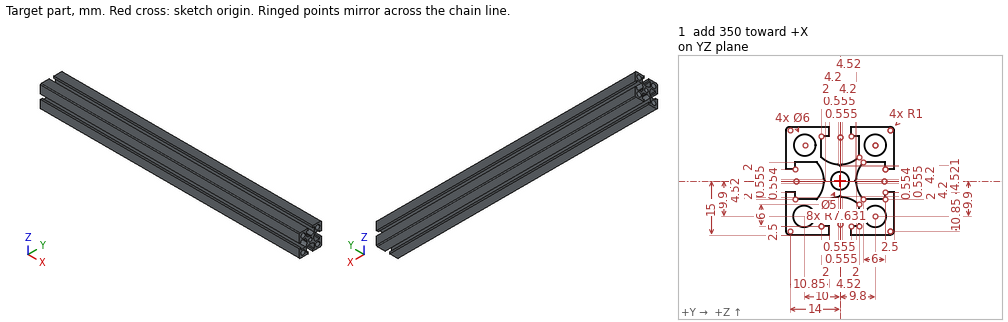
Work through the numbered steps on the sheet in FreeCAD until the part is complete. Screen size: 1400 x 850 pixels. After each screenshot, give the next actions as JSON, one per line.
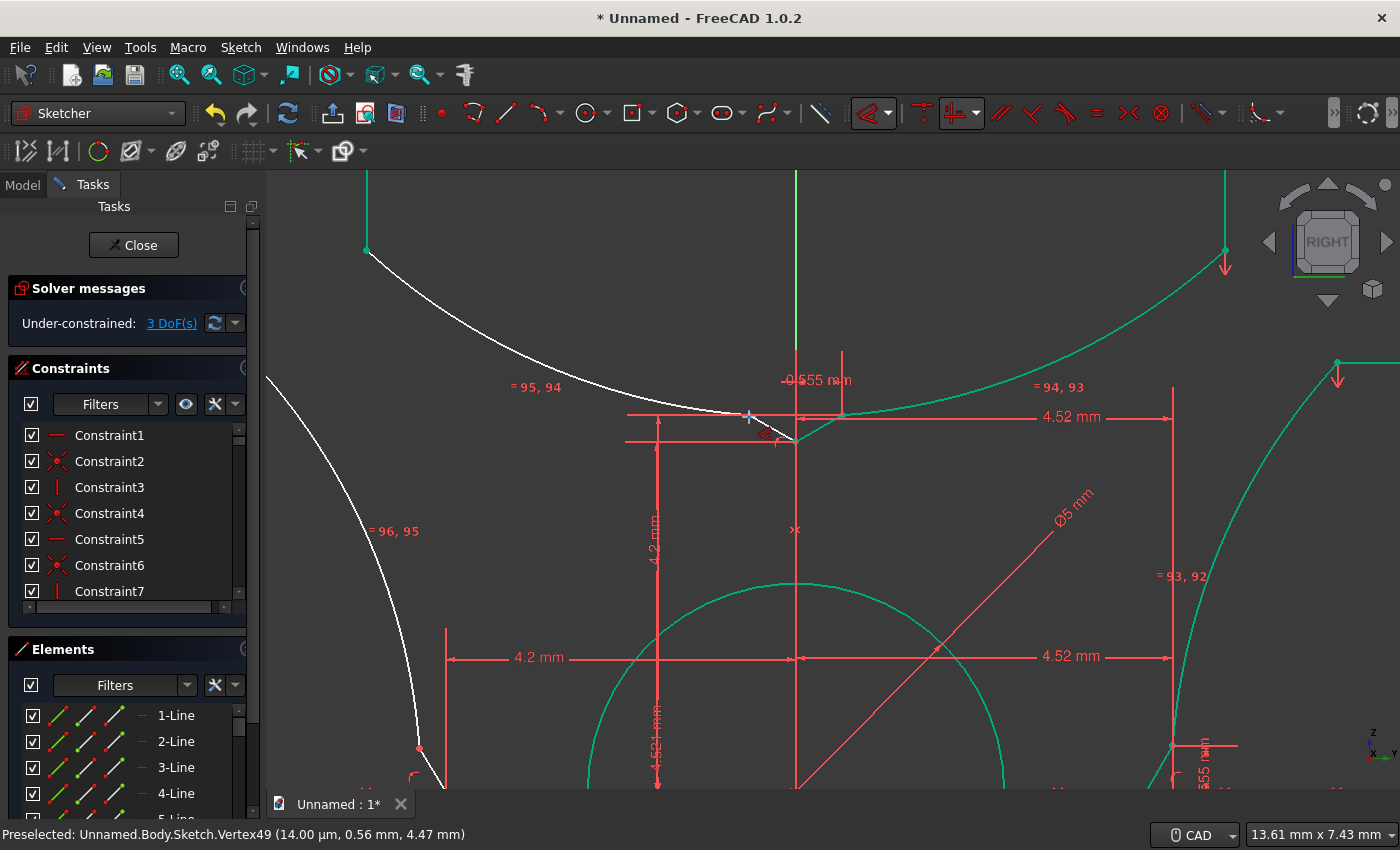
{"action": "left_click", "coordinate": [749, 415]}
{"action": "left_click", "coordinate": [773, 357]}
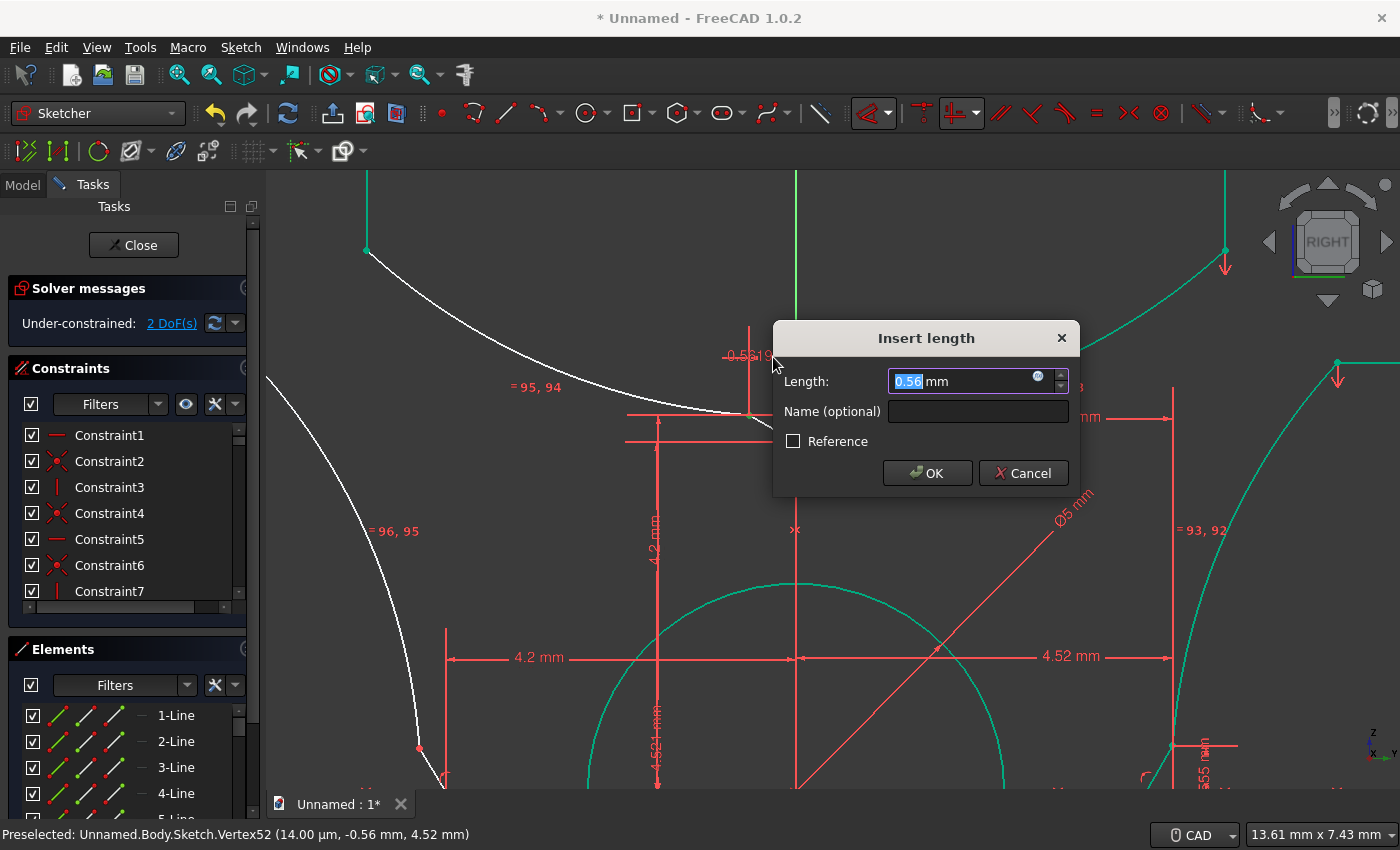
{"action": "type", "text": "0.555"}
{"action": "key", "text": "Return"}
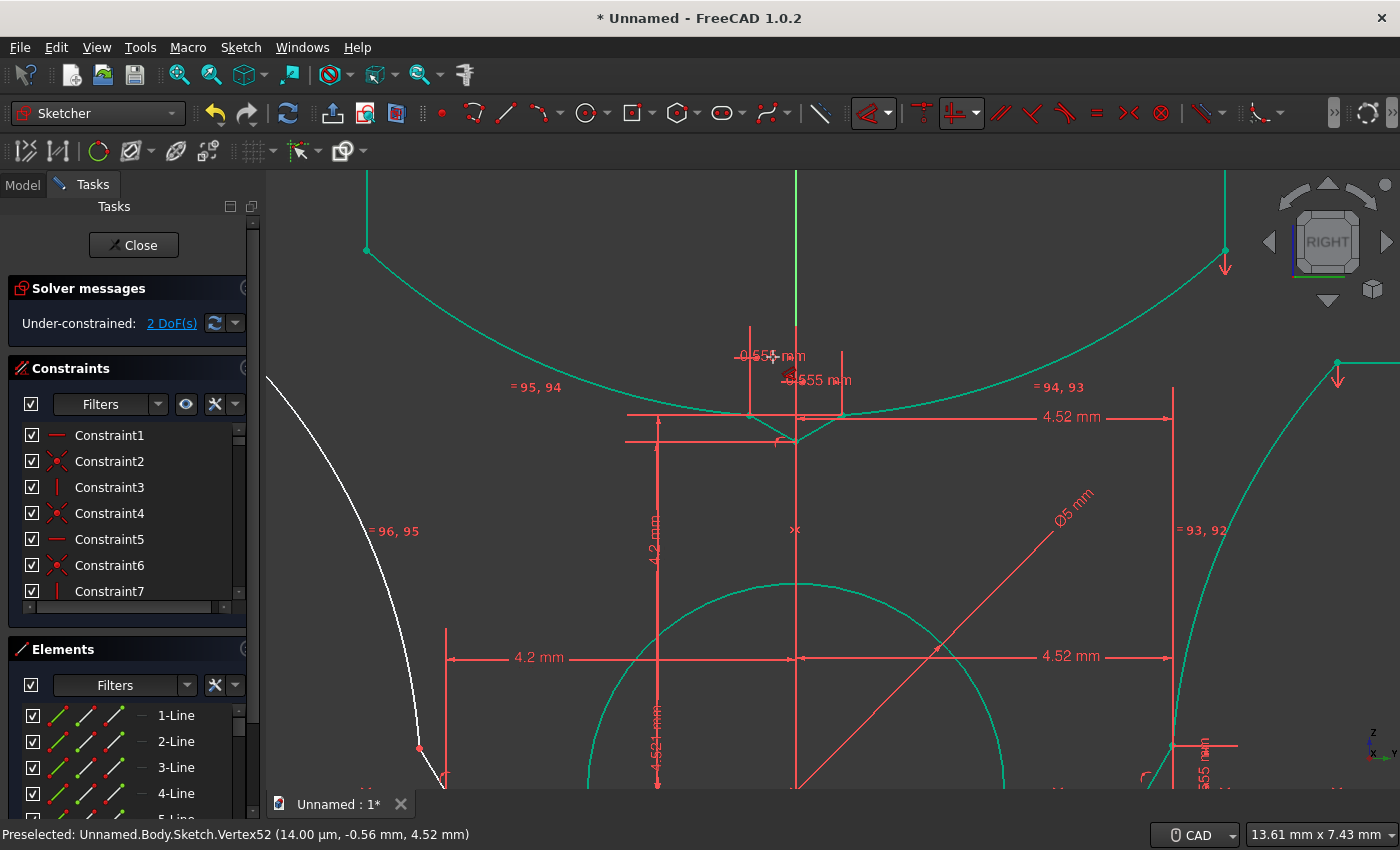
{"action": "left_click", "coordinate": [419, 748]}
{"action": "left_click", "coordinate": [385, 755]}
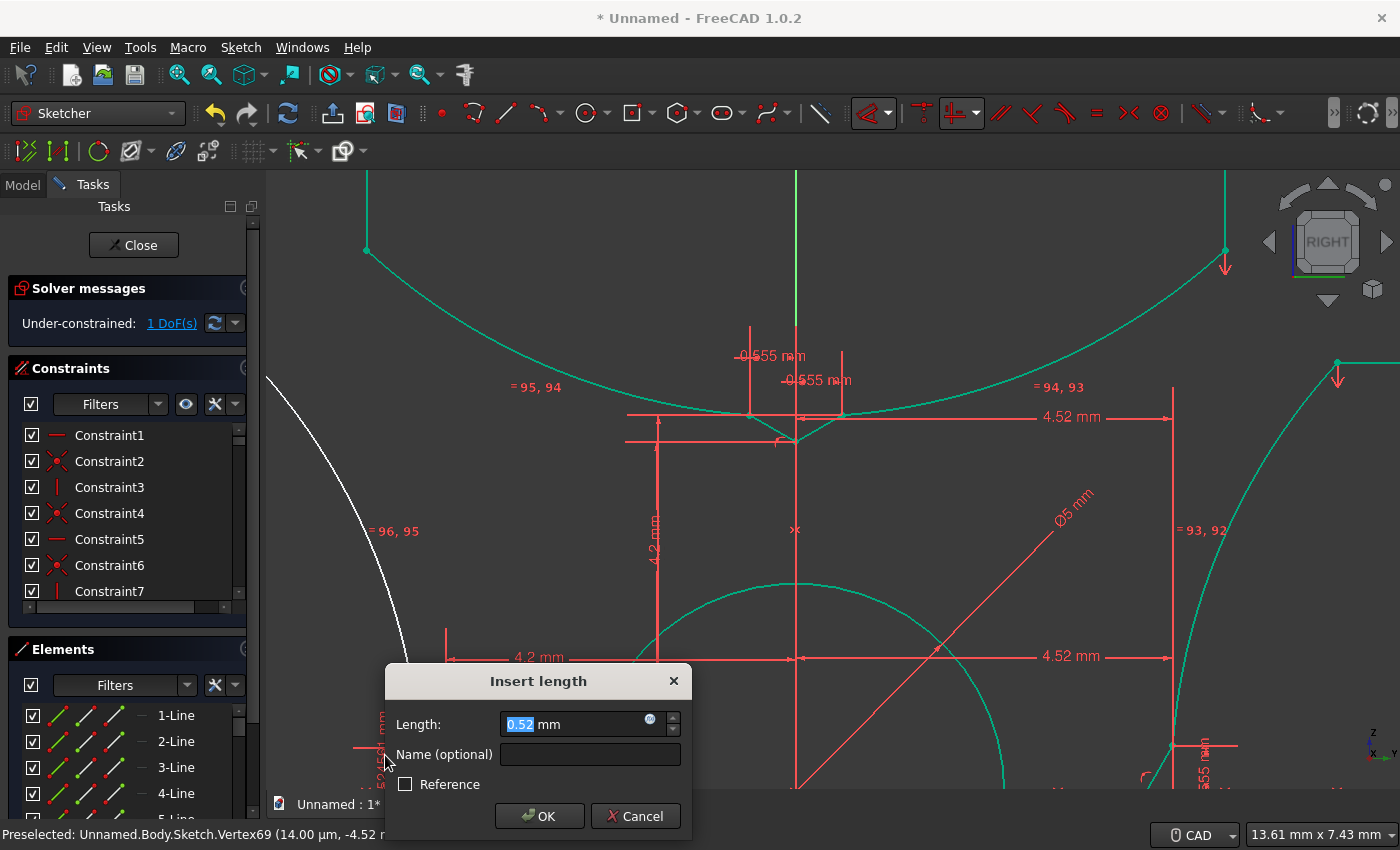
{"action": "type", "text": "0.555"}
{"action": "key", "text": "Return"}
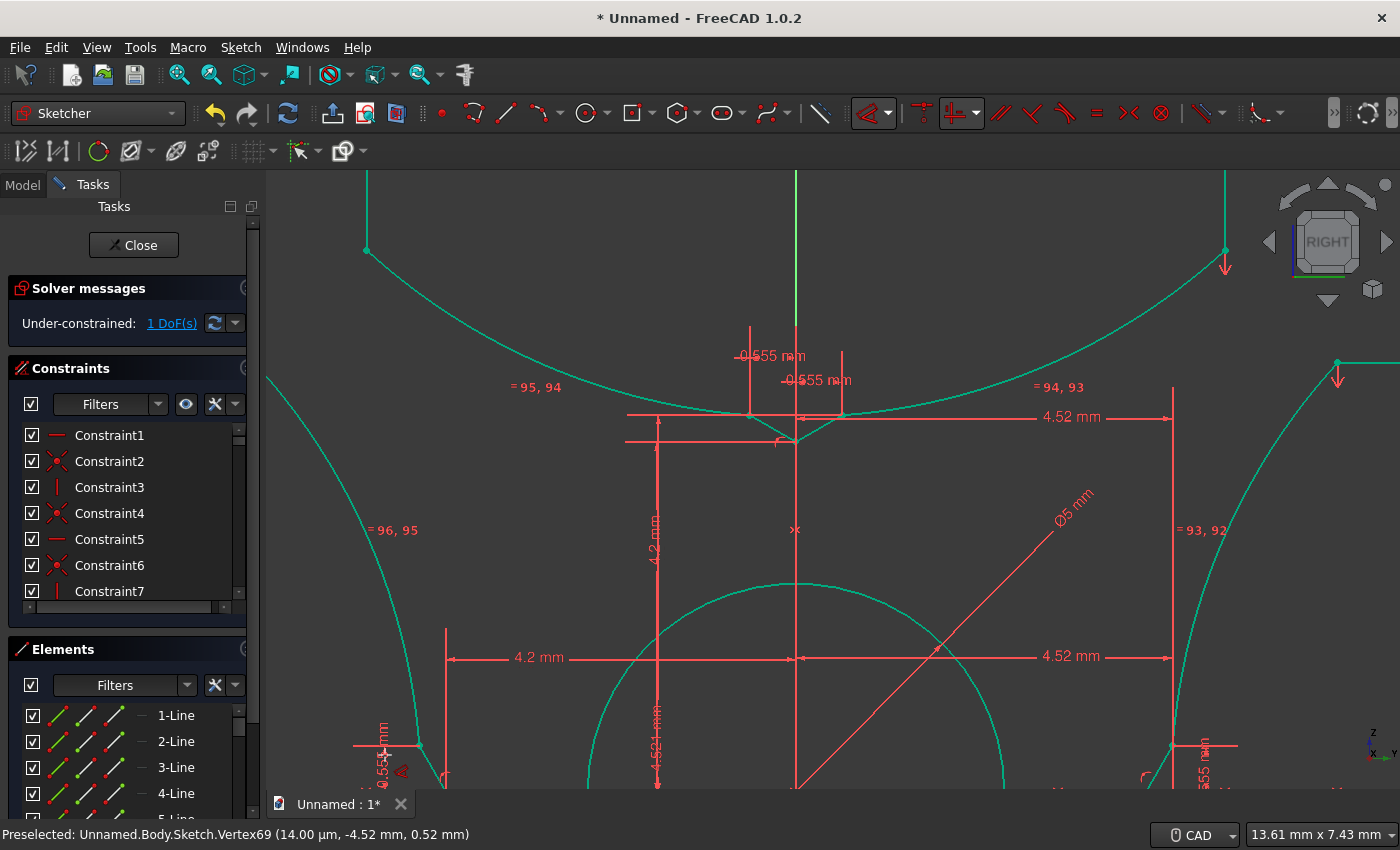
{"action": "scroll", "coordinate": [758, 418], "scroll_direction": "down", "scroll_amount": 9}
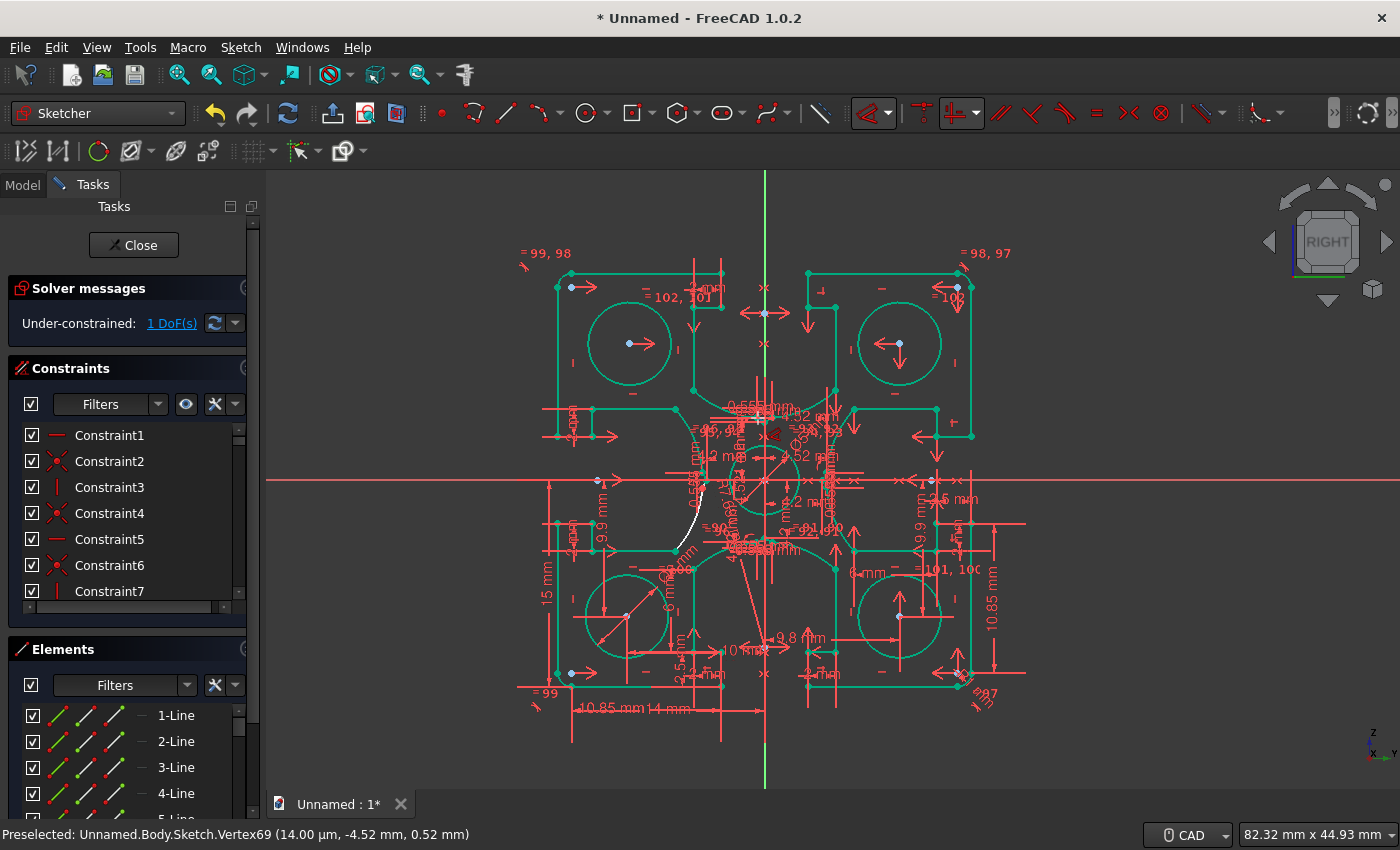
{"action": "scroll", "coordinate": [702, 488], "scroll_direction": "up", "scroll_amount": 9}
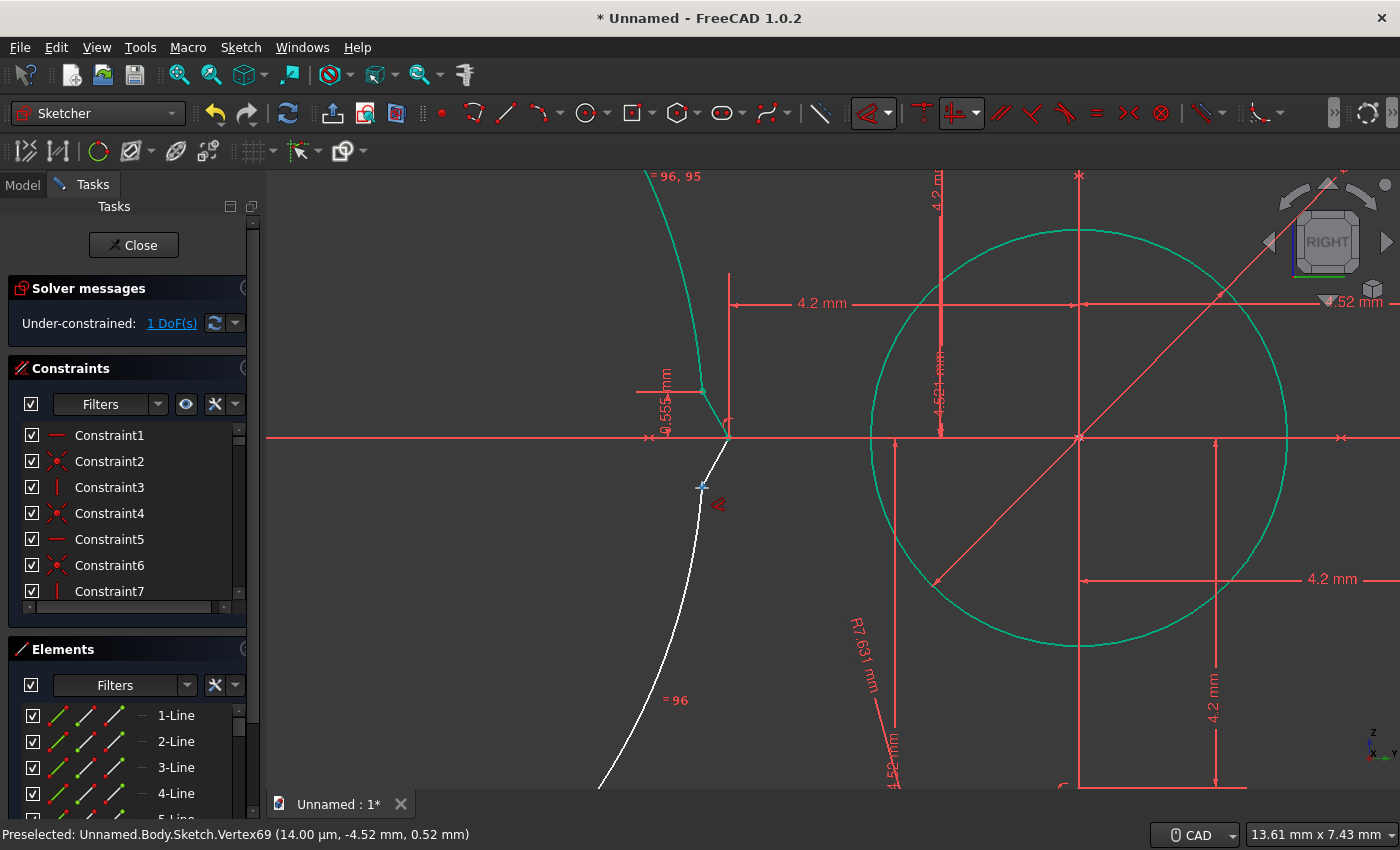
{"action": "left_click", "coordinate": [702, 487]}
{"action": "left_click", "coordinate": [668, 462]}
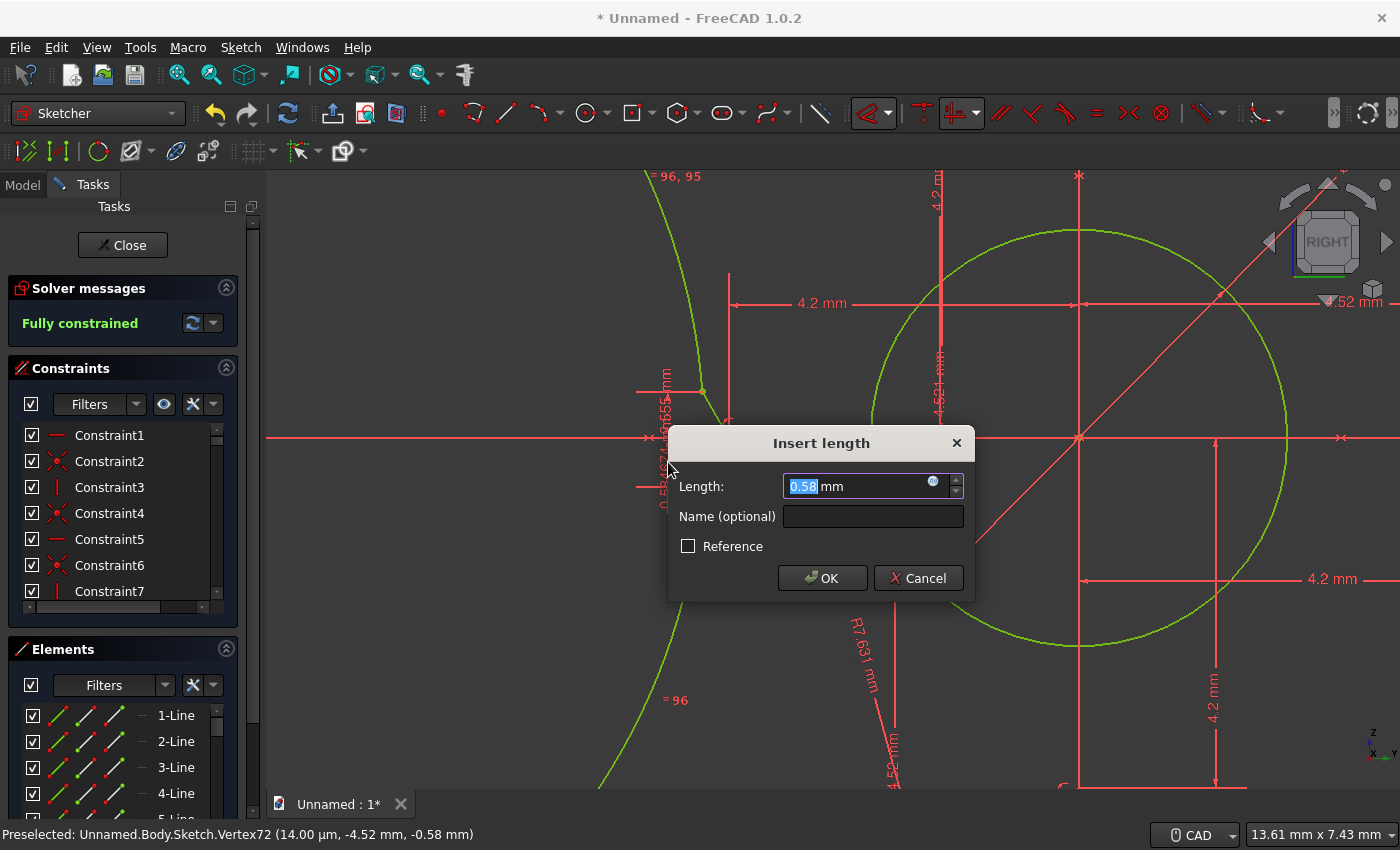
{"action": "type", "text": "0.554"}
{"action": "key", "text": "Return"}
{"action": "key", "text": "Escape"}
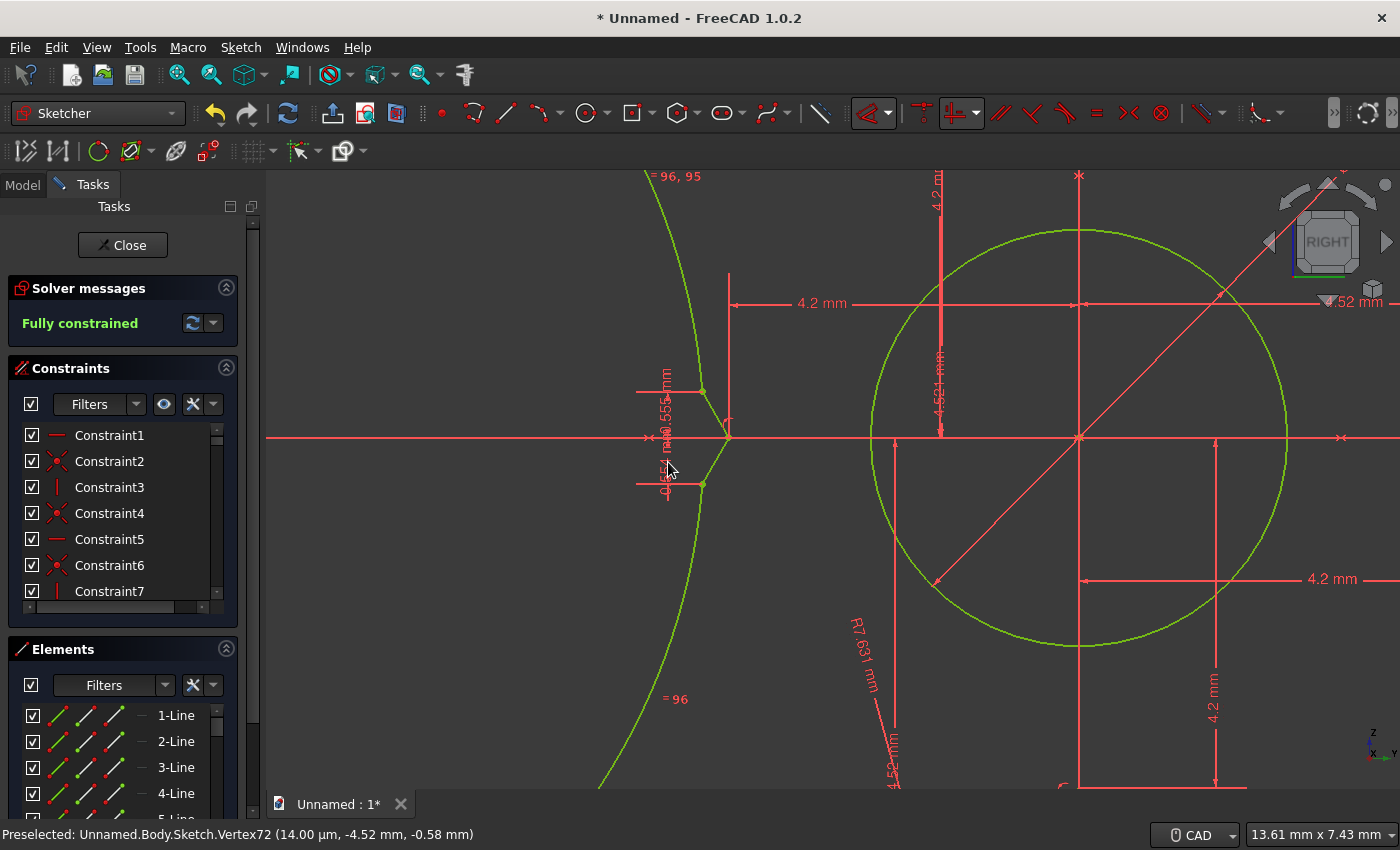
{"action": "left_click", "coordinate": [123, 245]}